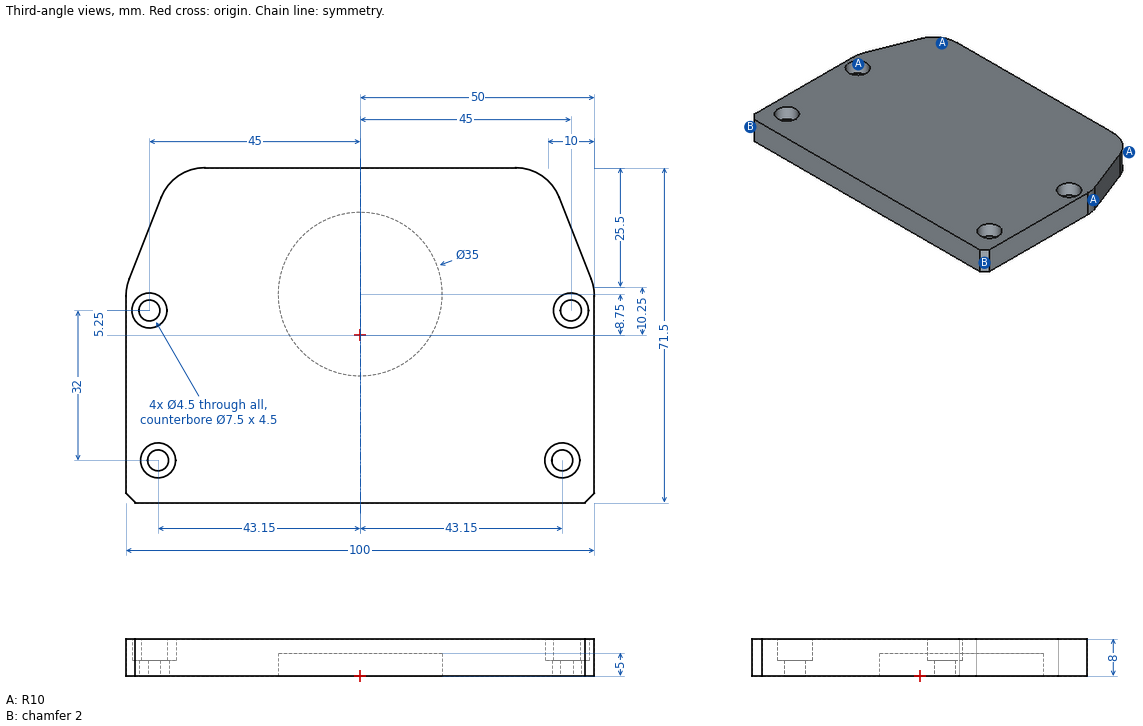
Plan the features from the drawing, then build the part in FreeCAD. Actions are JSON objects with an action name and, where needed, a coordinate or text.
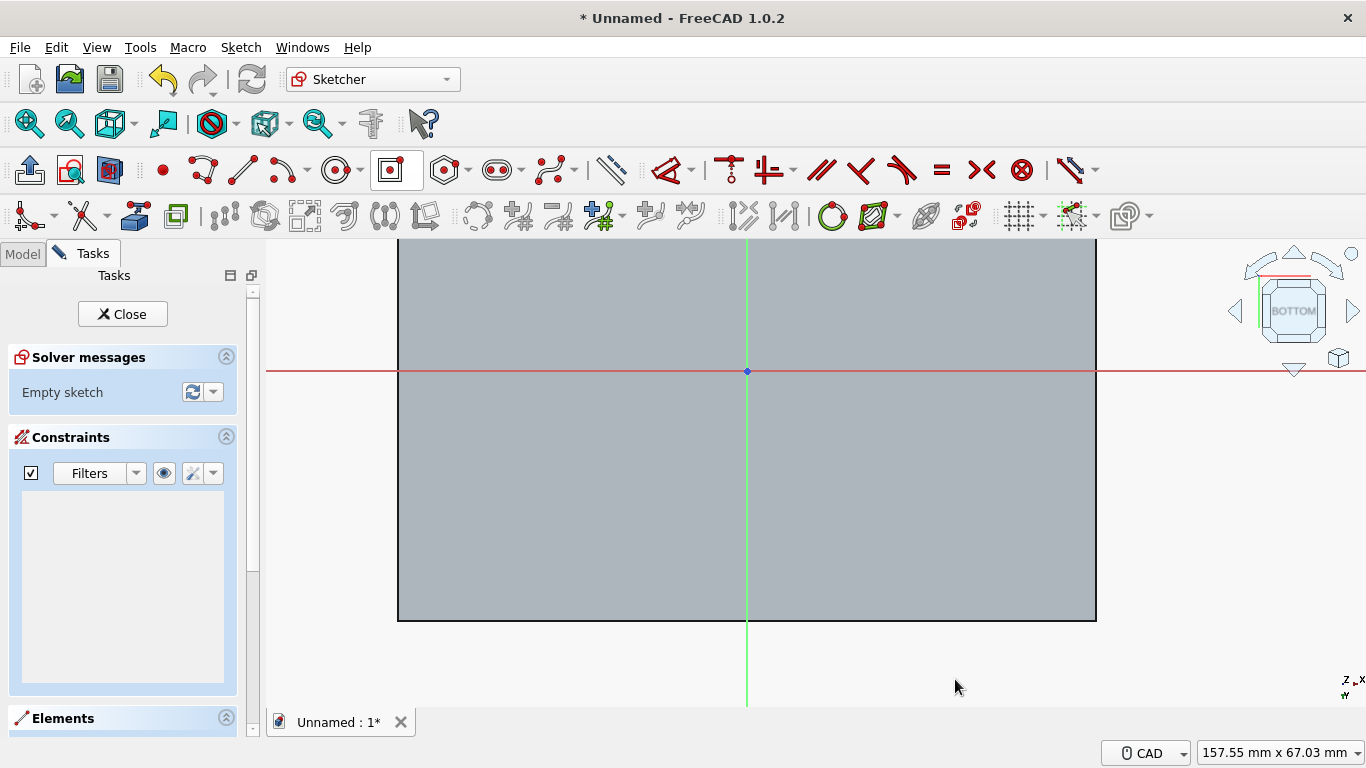
{"action": "left_click", "coordinate": [204, 170]}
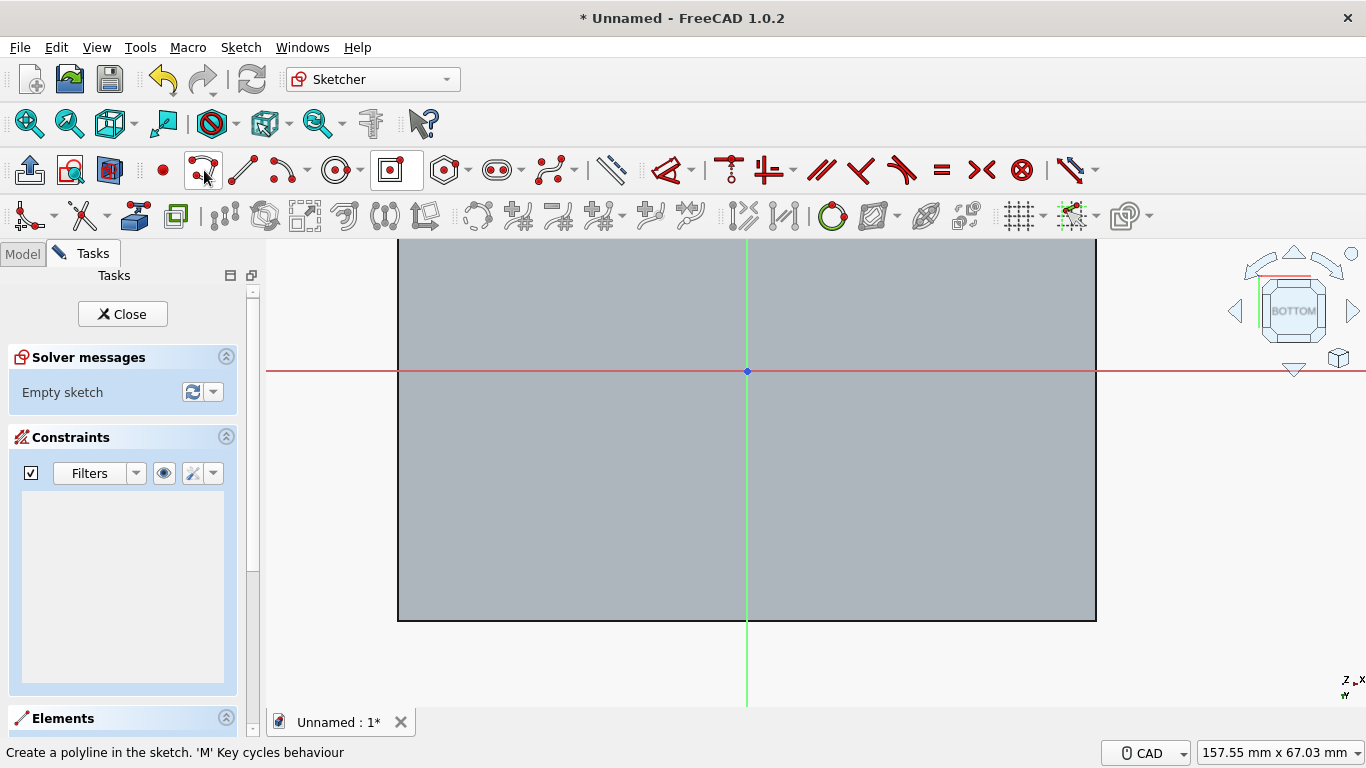
{"action": "left_click", "coordinate": [1096, 443]}
{"action": "left_click", "coordinate": [1027, 621]}
{"action": "left_click", "coordinate": [1096, 621]}
{"action": "left_click", "coordinate": [1096, 444]}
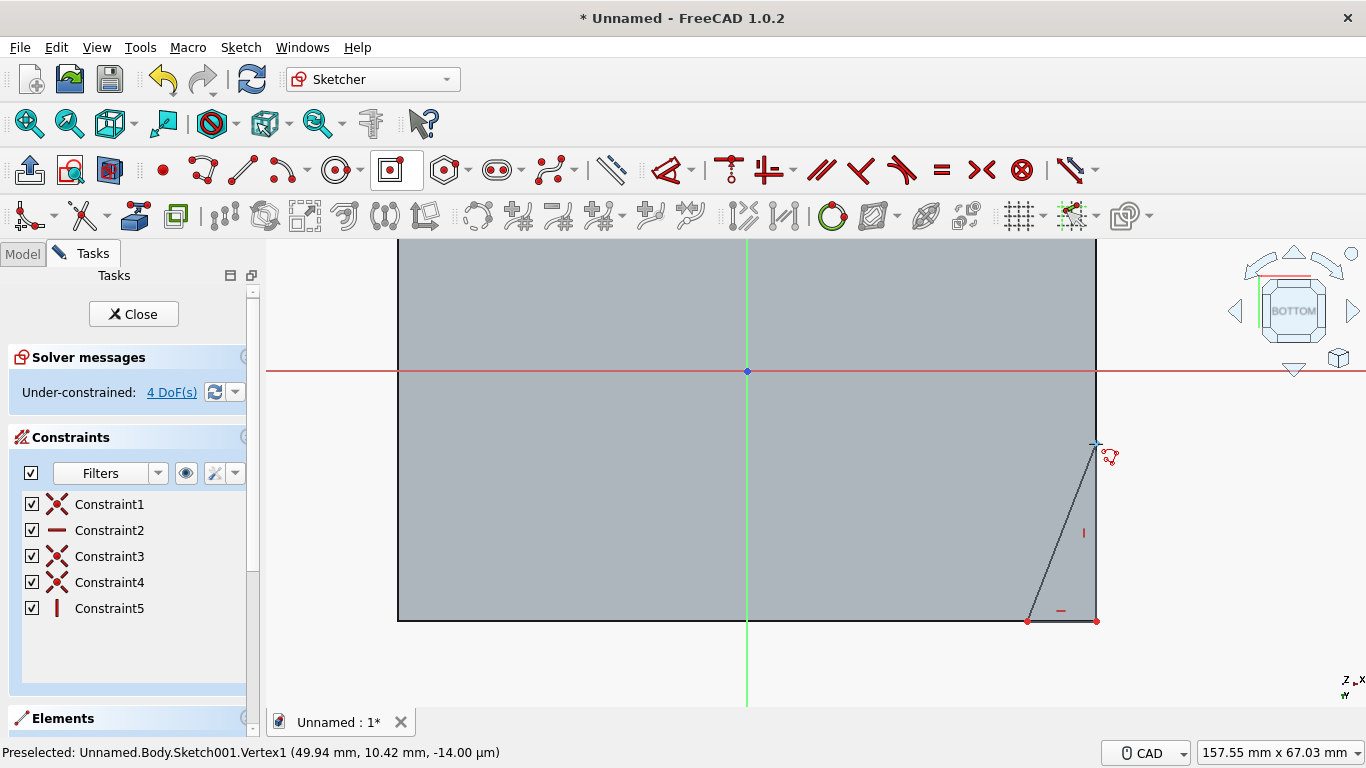
{"action": "left_click", "coordinate": [398, 443]}
{"action": "left_click", "coordinate": [398, 621]}
{"action": "left_click", "coordinate": [468, 621]}
{"action": "left_click", "coordinate": [398, 444]}
{"action": "key", "text": "Escape"}
{"action": "key", "text": "Escape"}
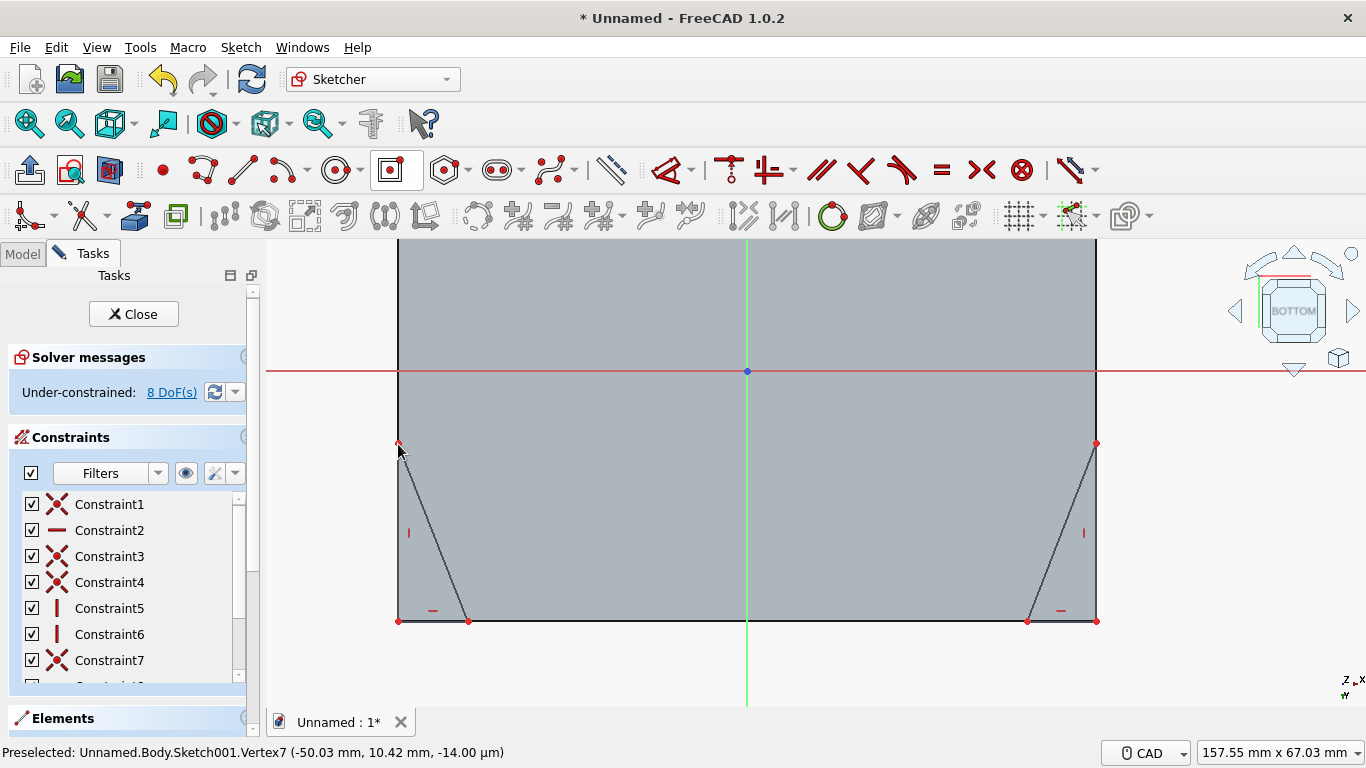
{"action": "left_click", "coordinate": [1096, 444]}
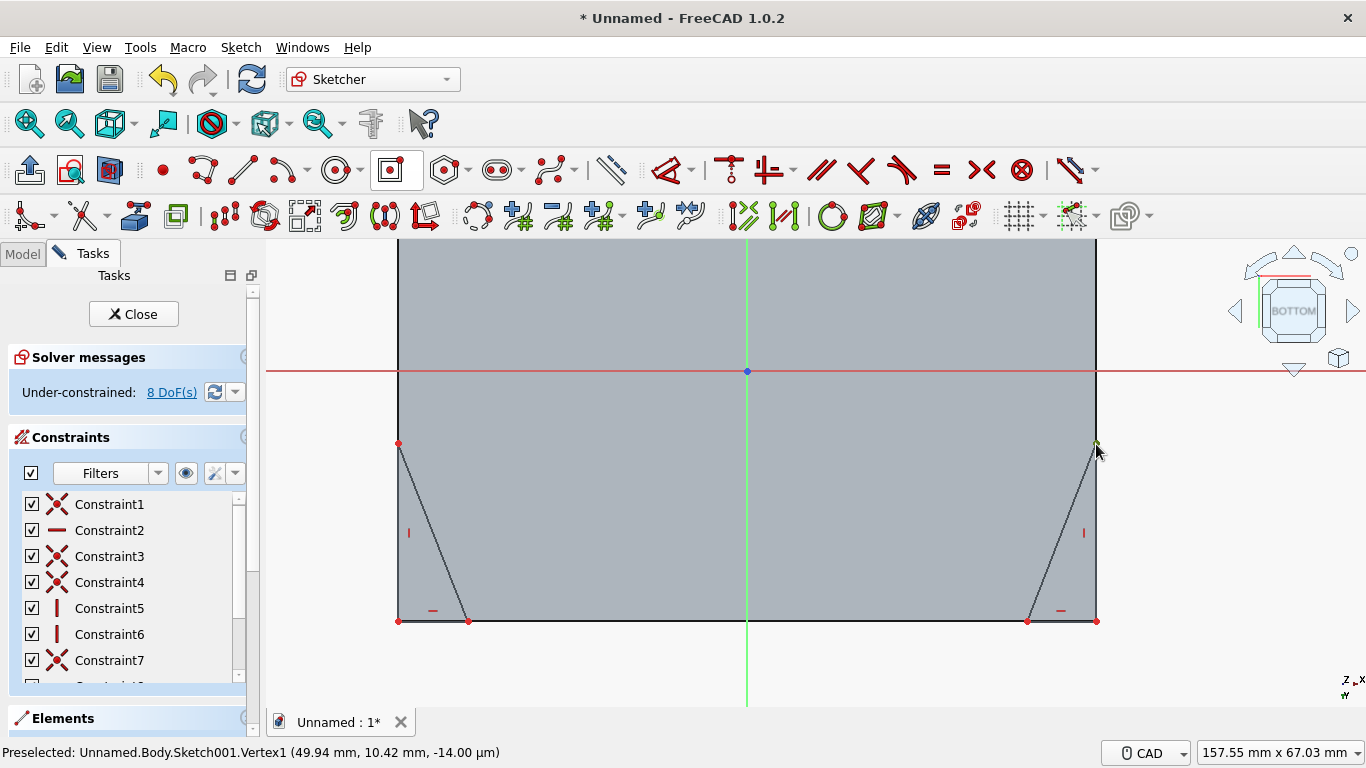
{"action": "left_click", "coordinate": [398, 444]}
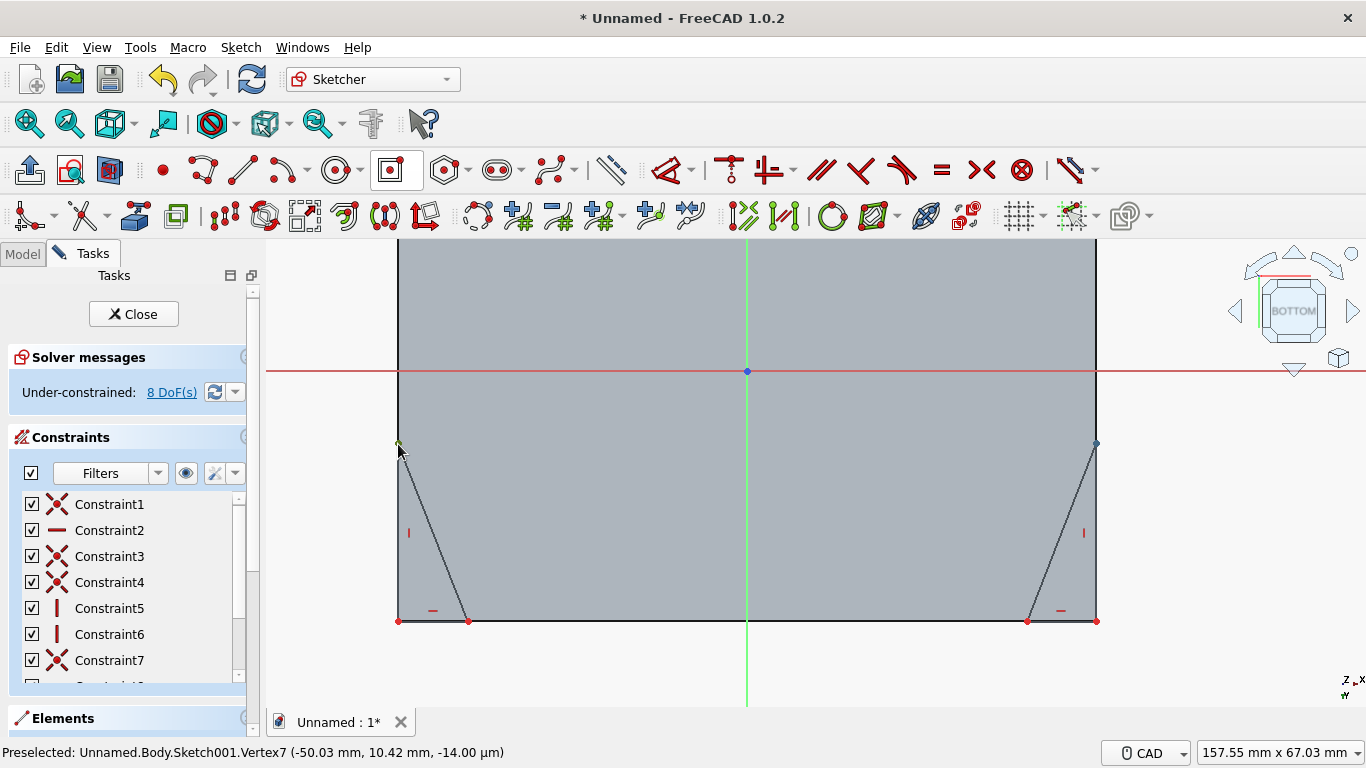
{"action": "left_click", "coordinate": [747, 650]}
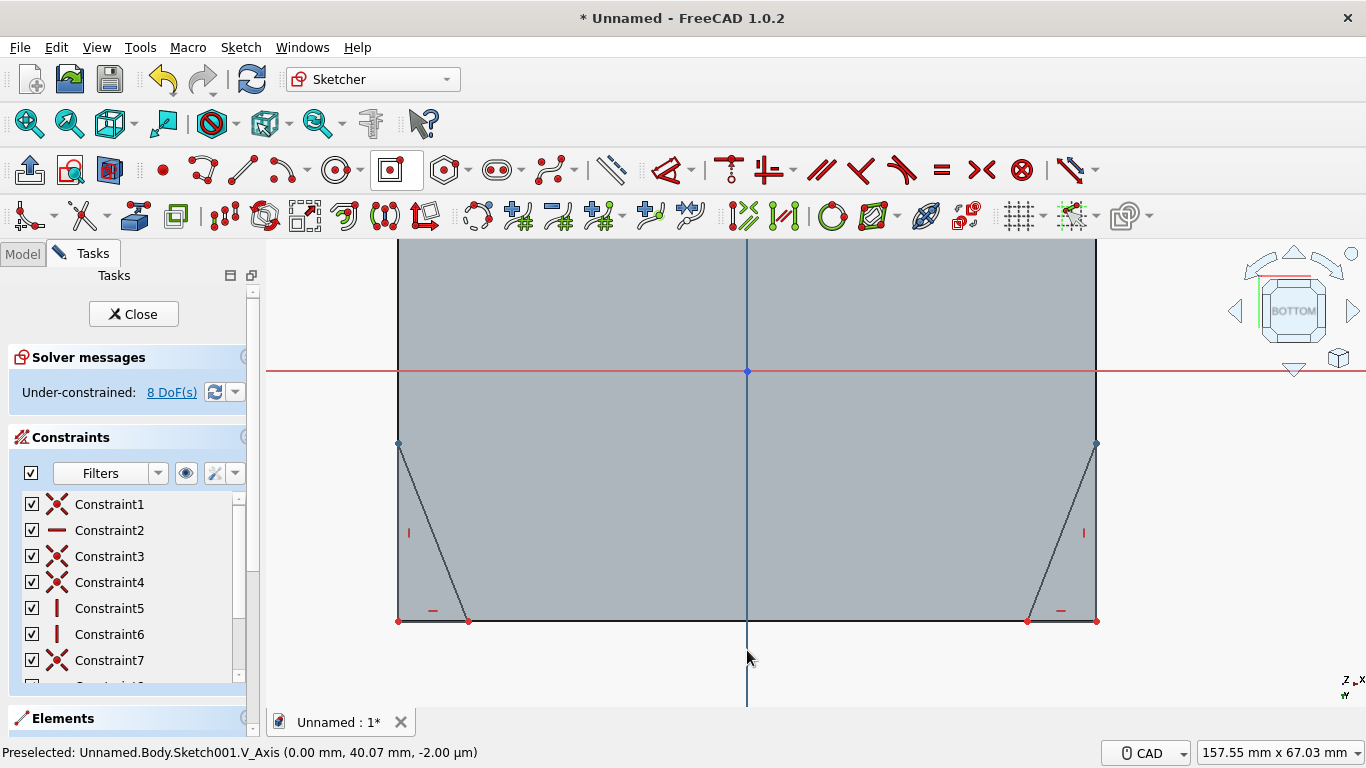
{"action": "left_click", "coordinate": [982, 170]}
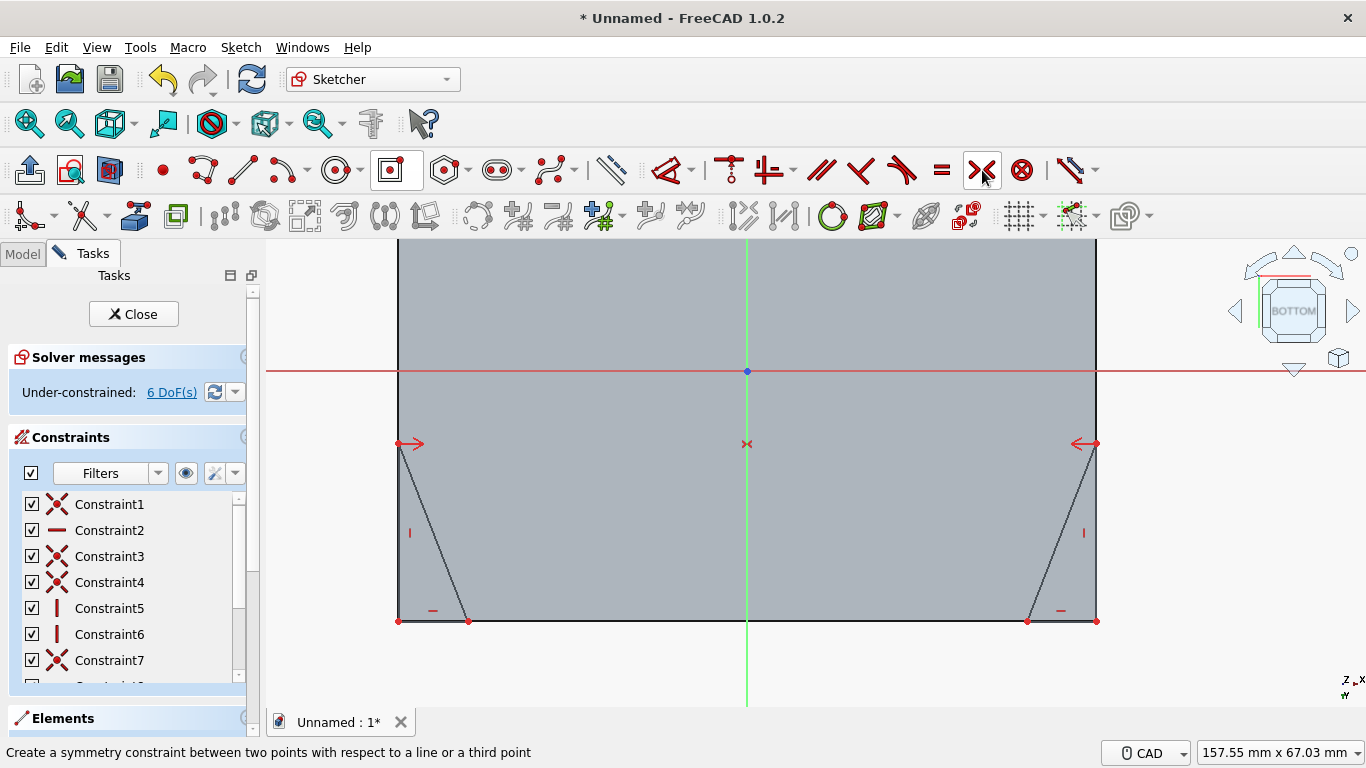
{"action": "left_click", "coordinate": [1027, 622]}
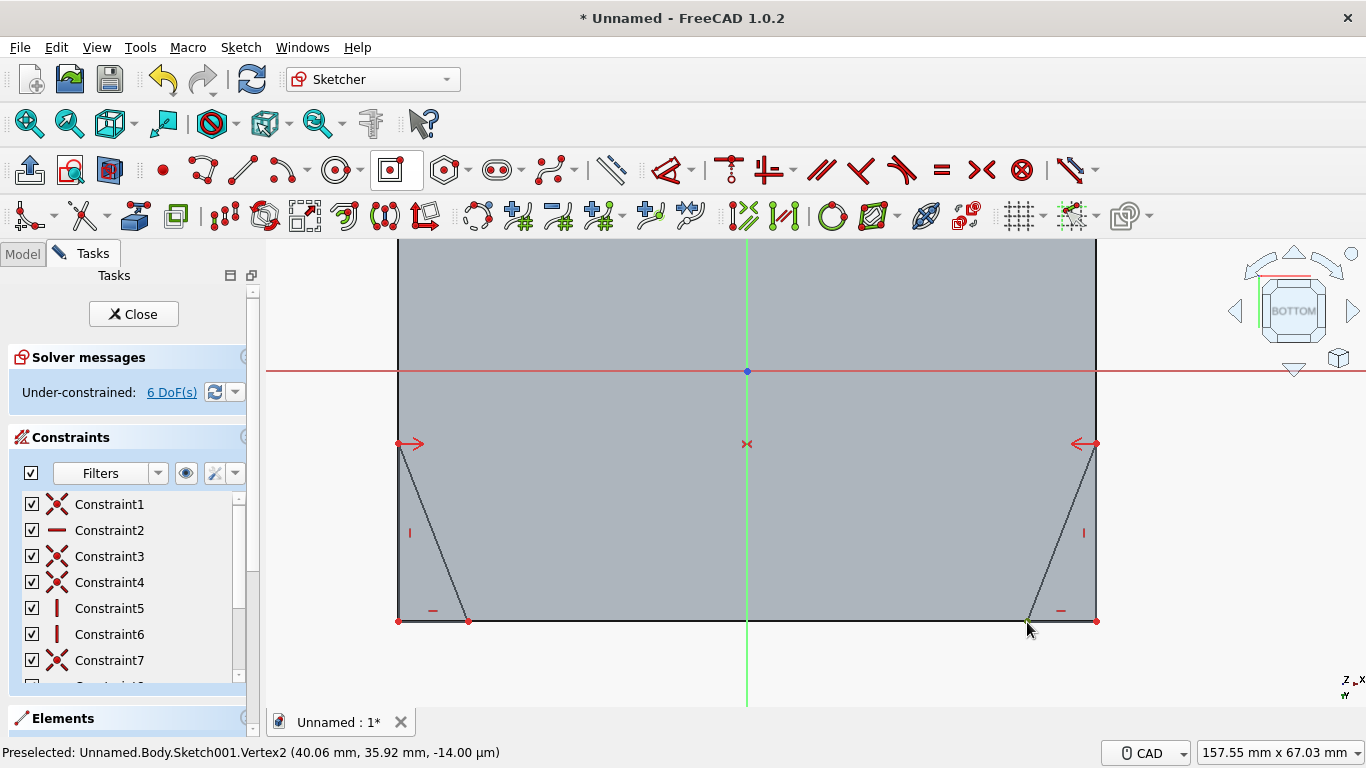
{"action": "left_click", "coordinate": [468, 622]}